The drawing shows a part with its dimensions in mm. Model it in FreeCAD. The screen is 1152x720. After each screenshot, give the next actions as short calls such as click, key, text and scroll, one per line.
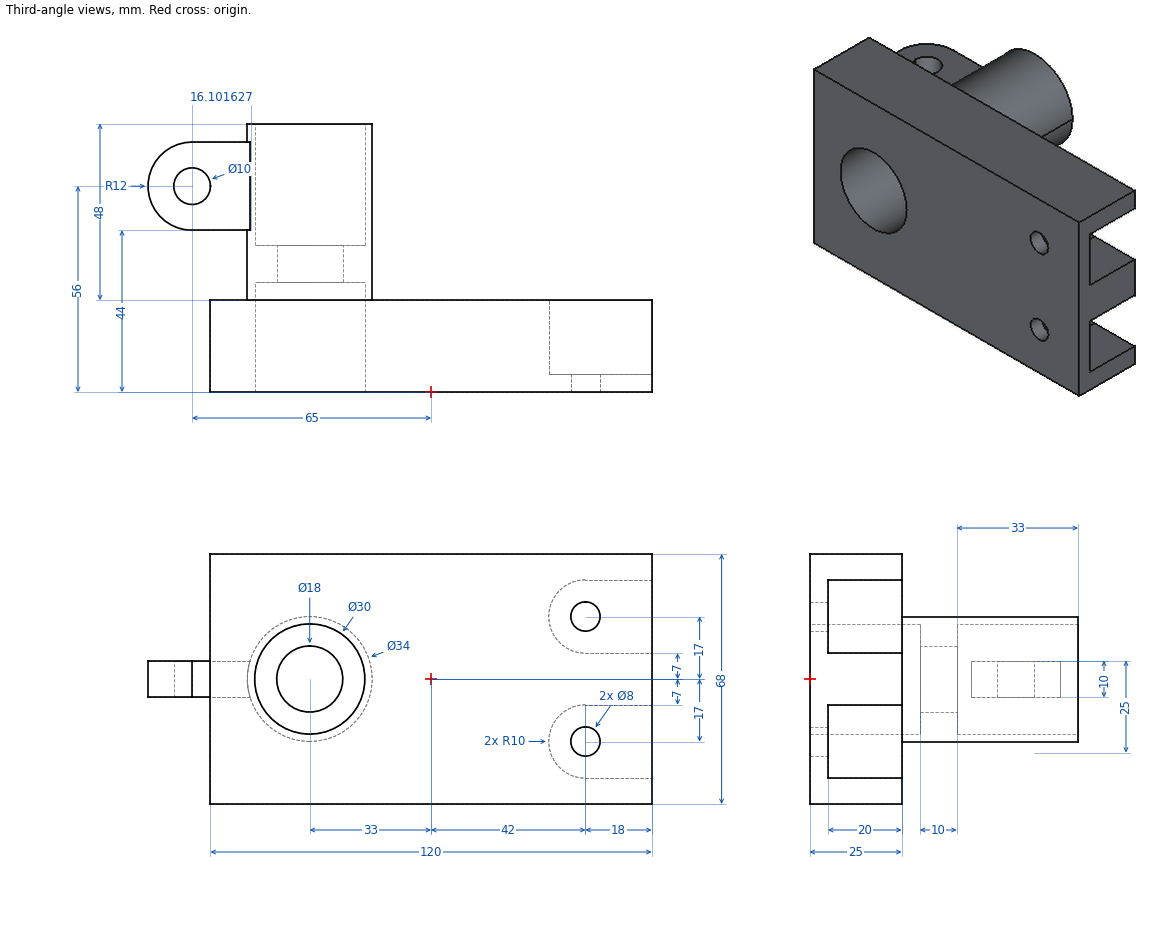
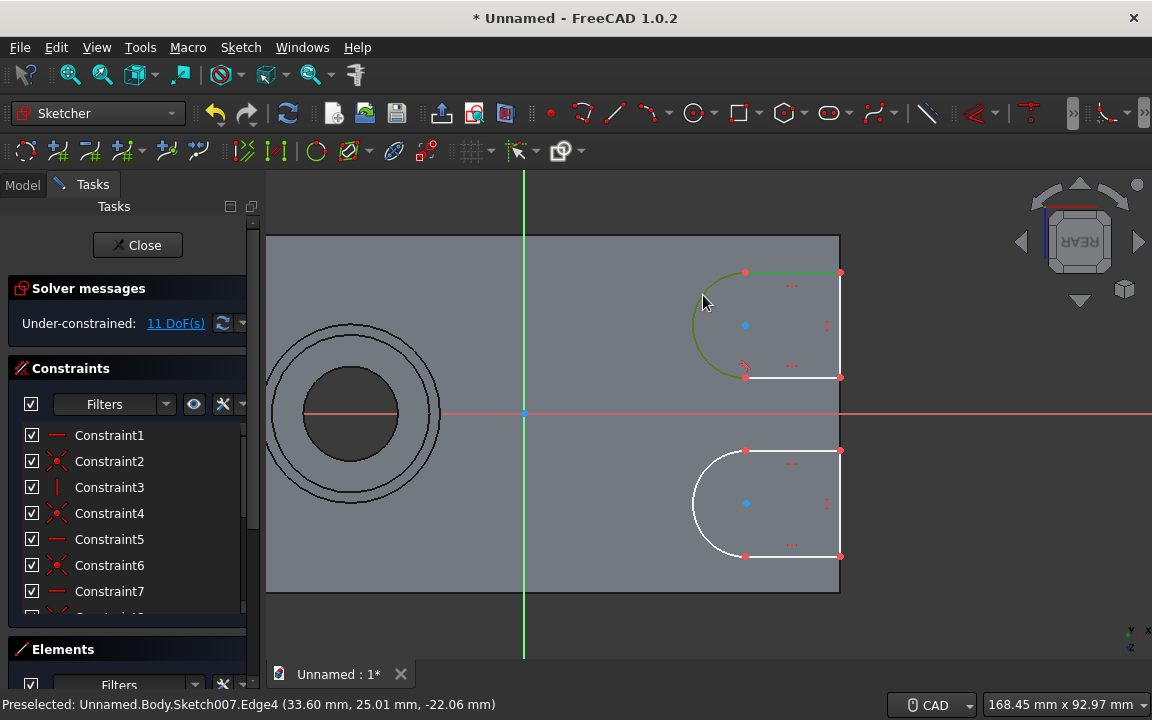
key(t)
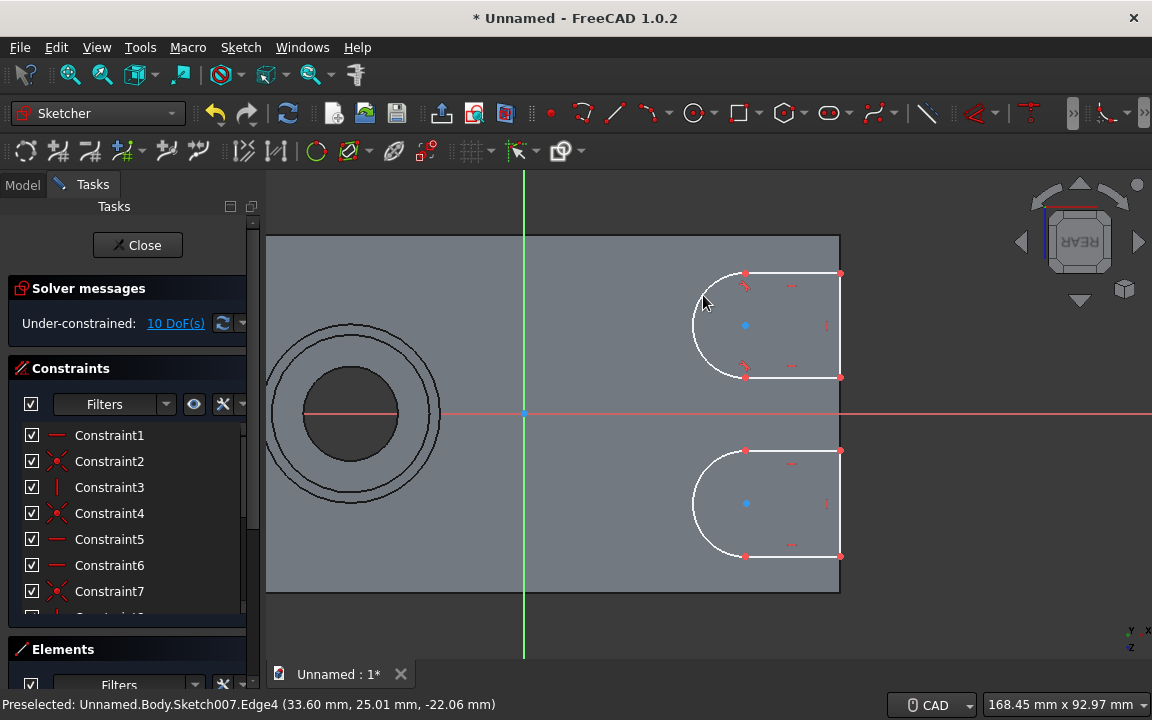
click(774, 557)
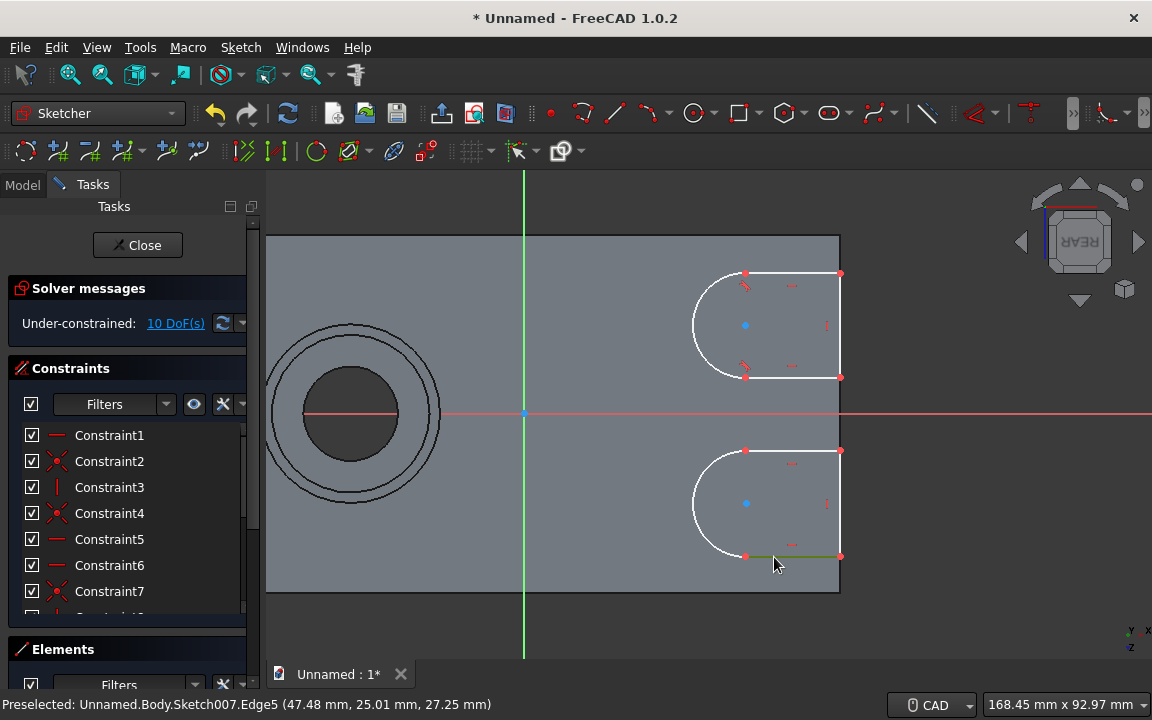
click(703, 473)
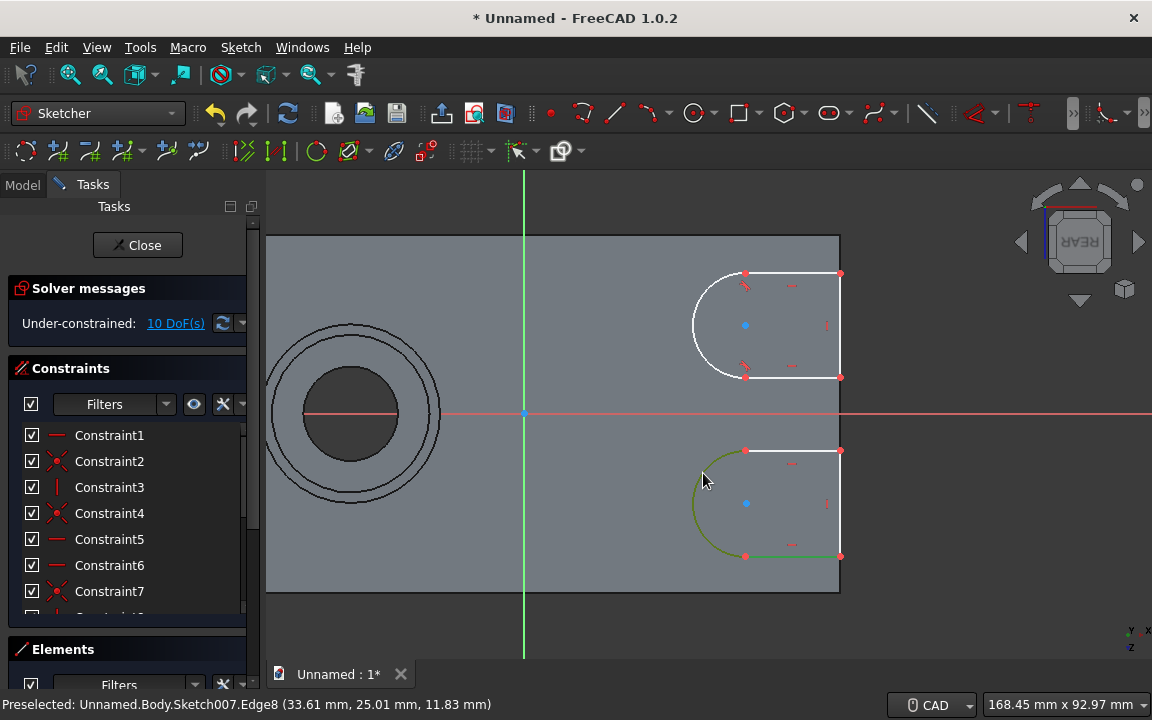
key(t)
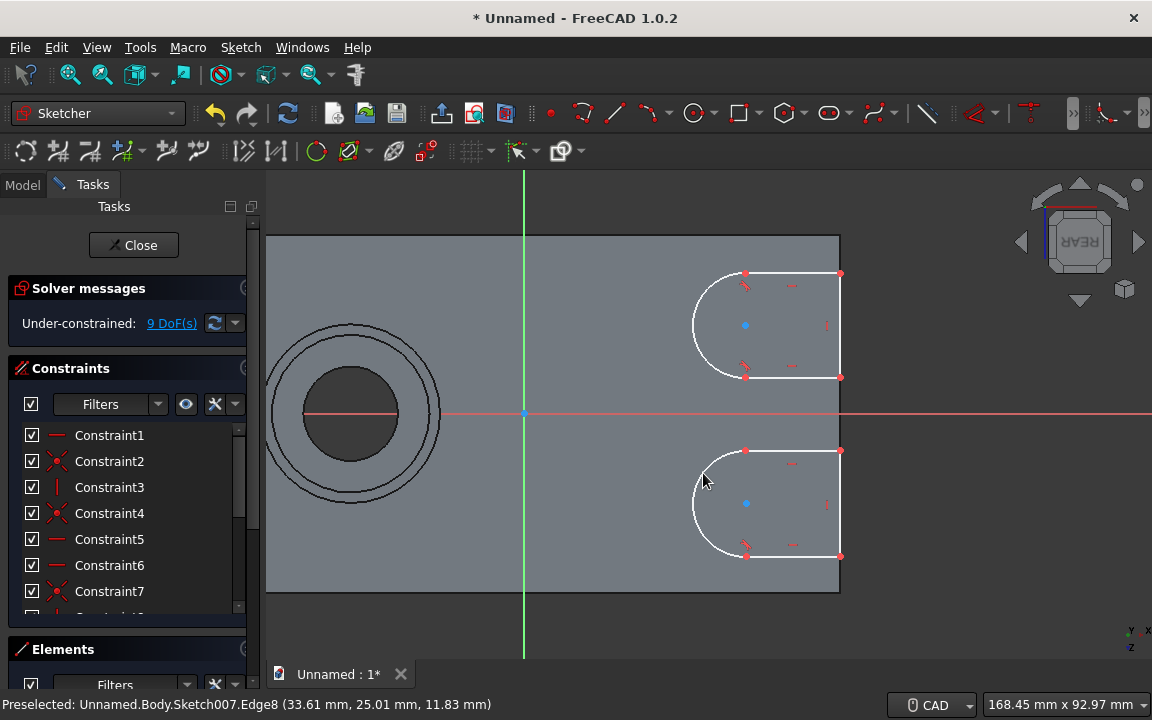
click(812, 451)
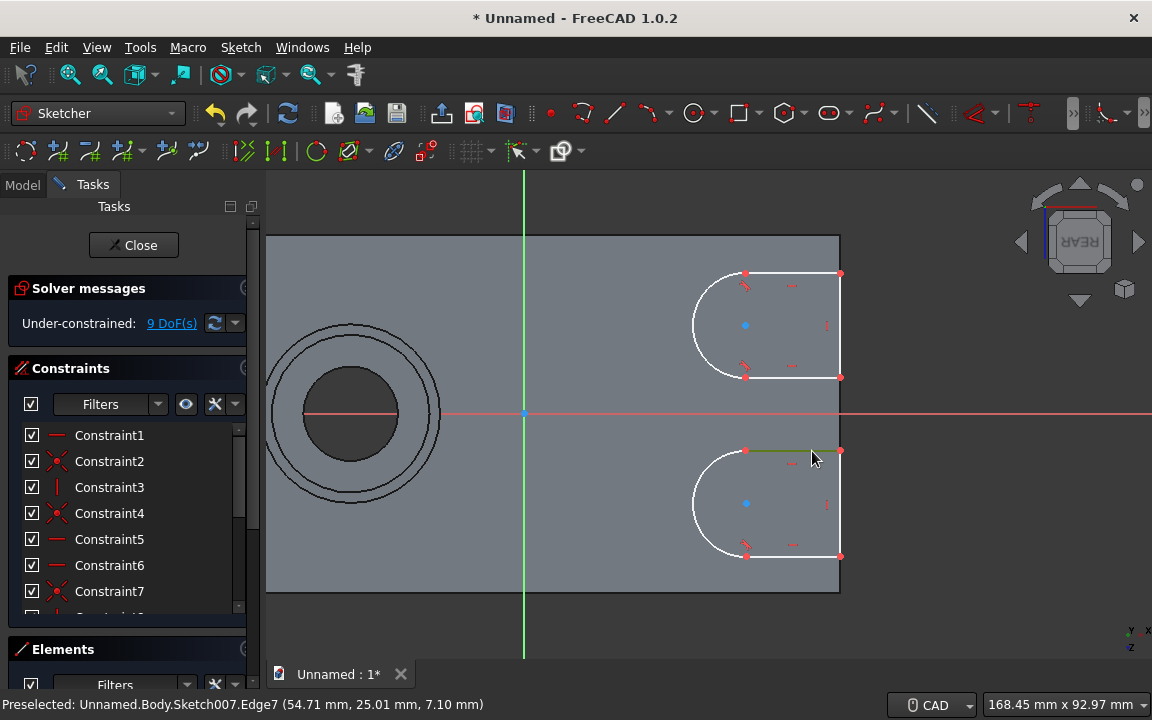
click(703, 473)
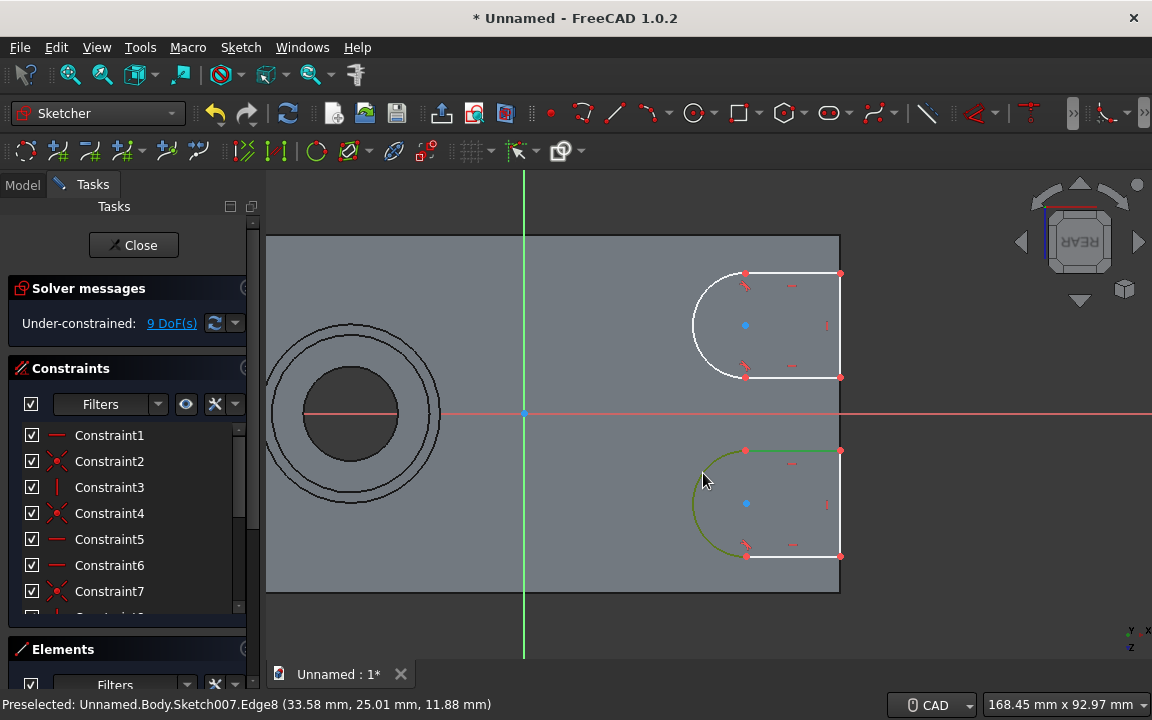
key(t)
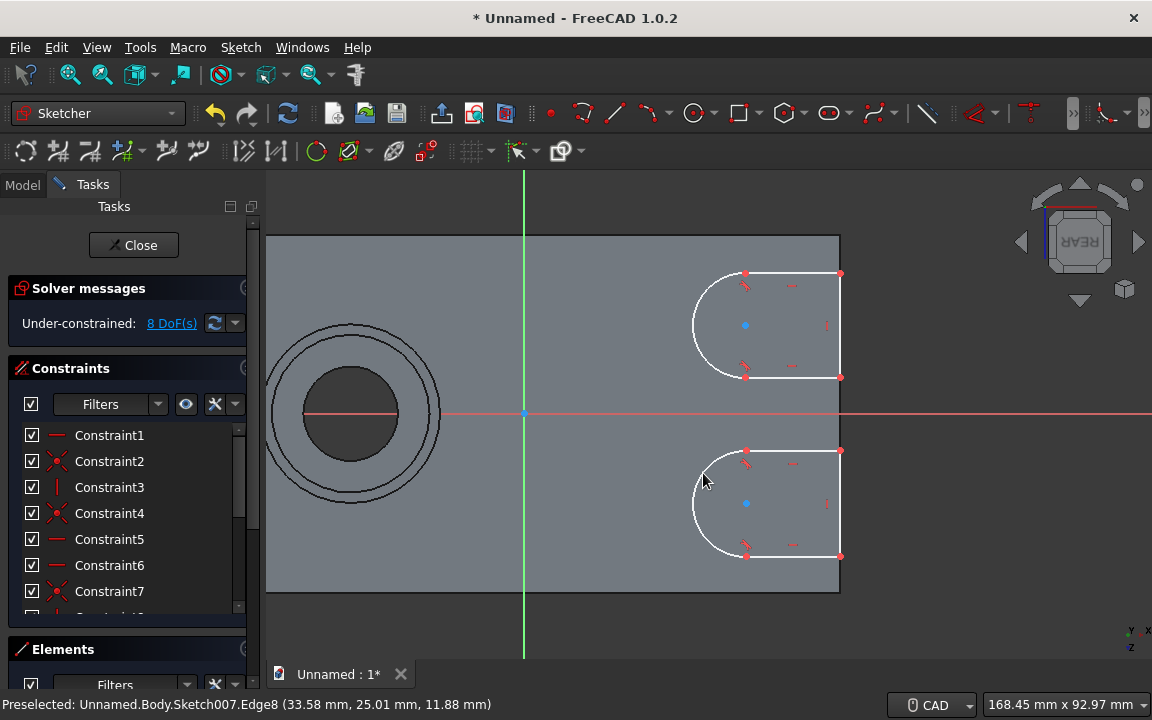
click(703, 295)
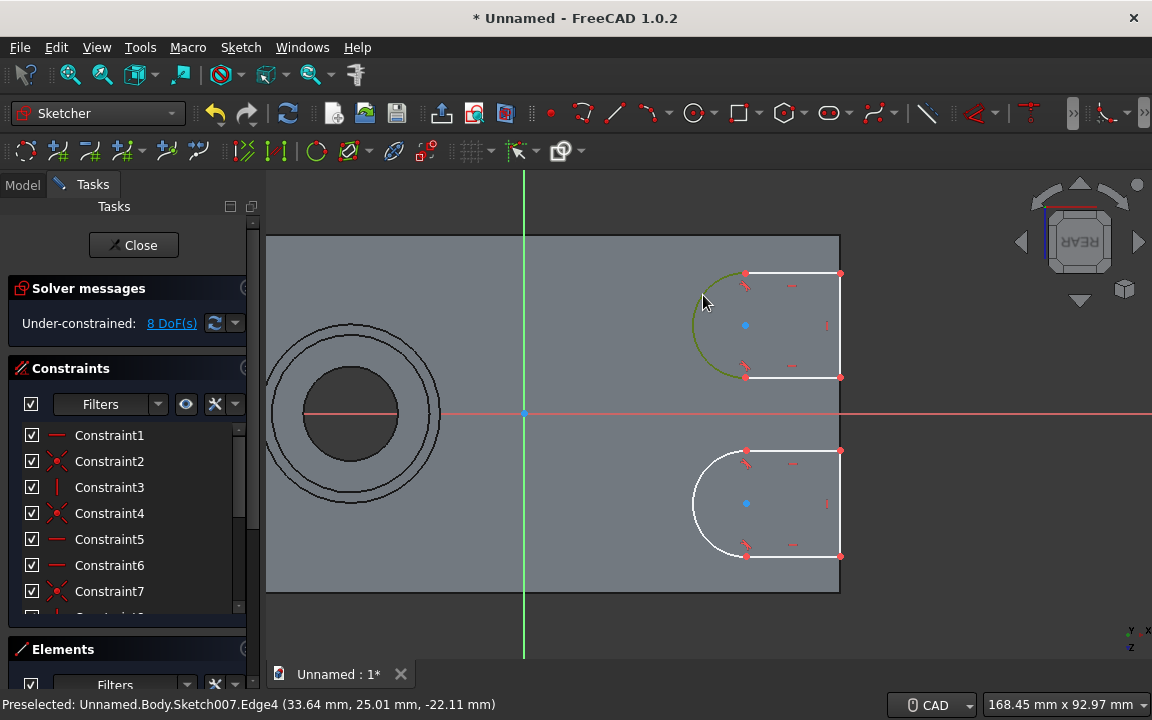
click(703, 473)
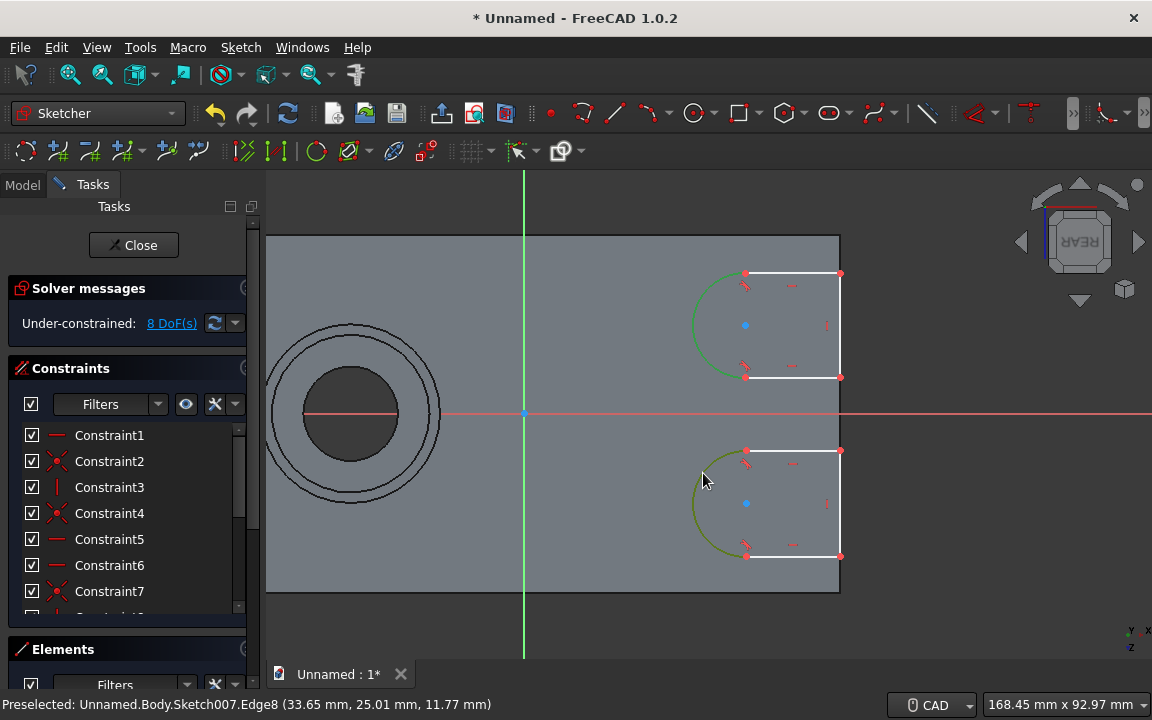
key(e)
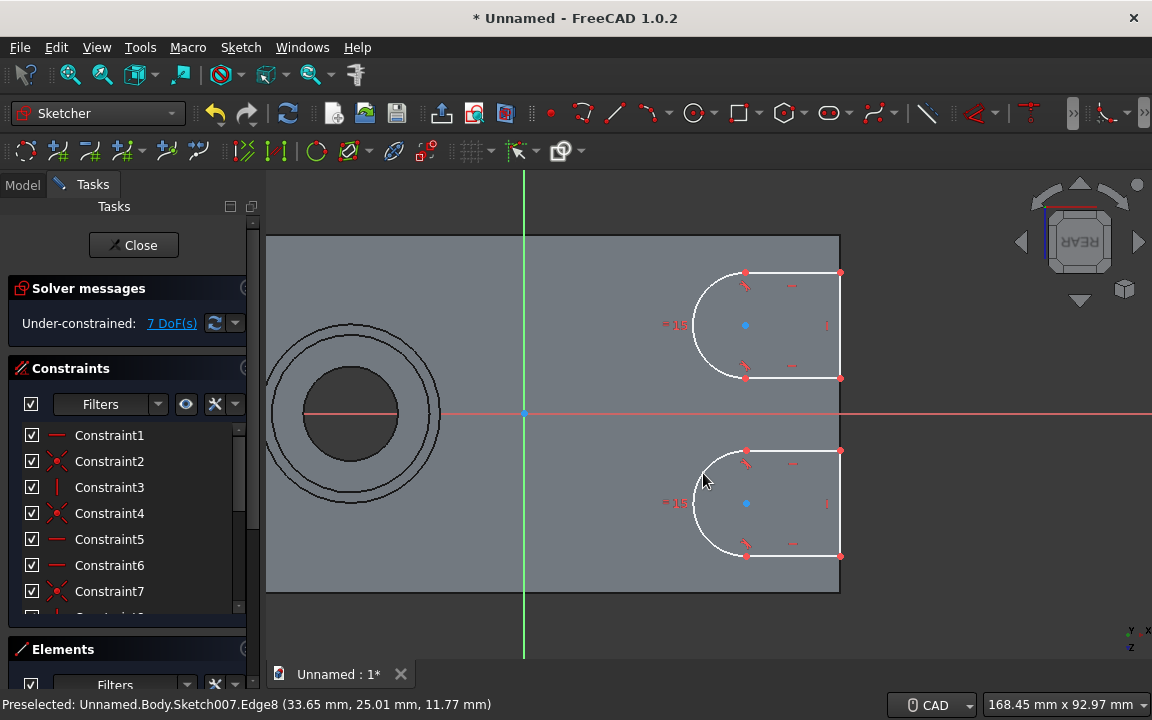
click(974, 114)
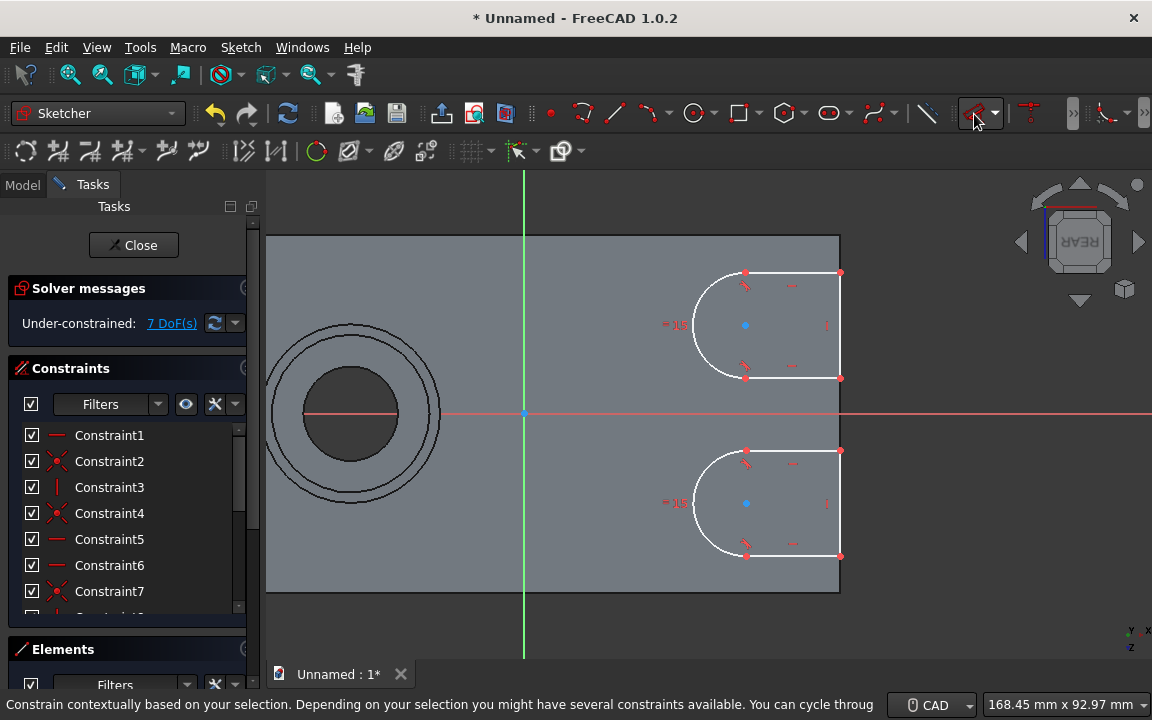
click(703, 295)
click(677, 276)